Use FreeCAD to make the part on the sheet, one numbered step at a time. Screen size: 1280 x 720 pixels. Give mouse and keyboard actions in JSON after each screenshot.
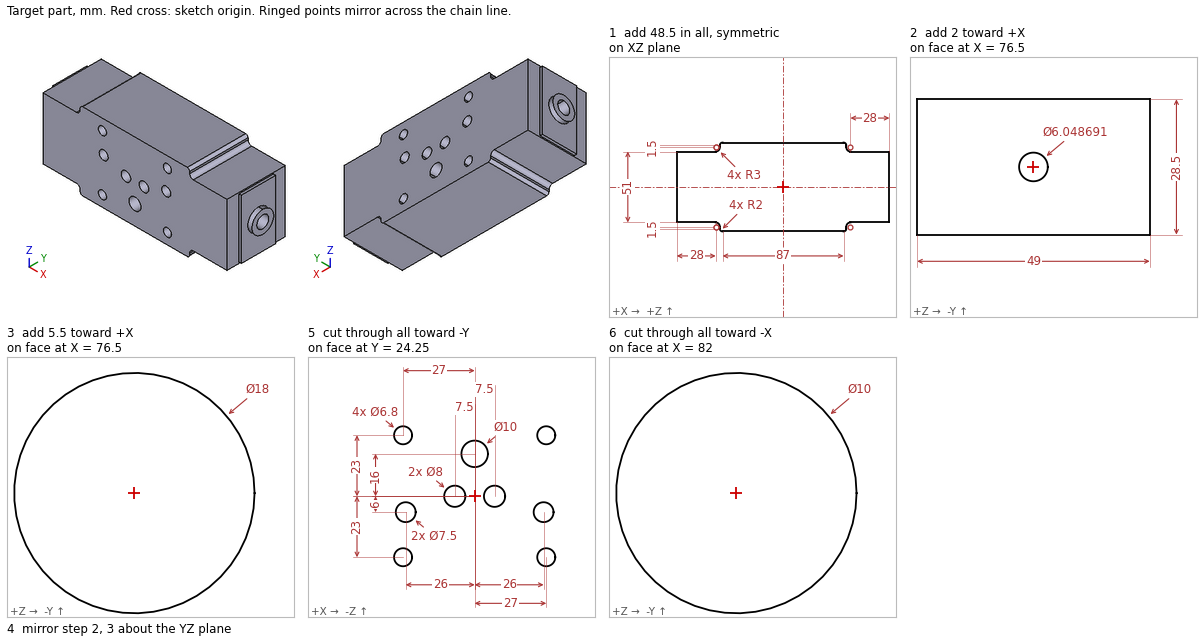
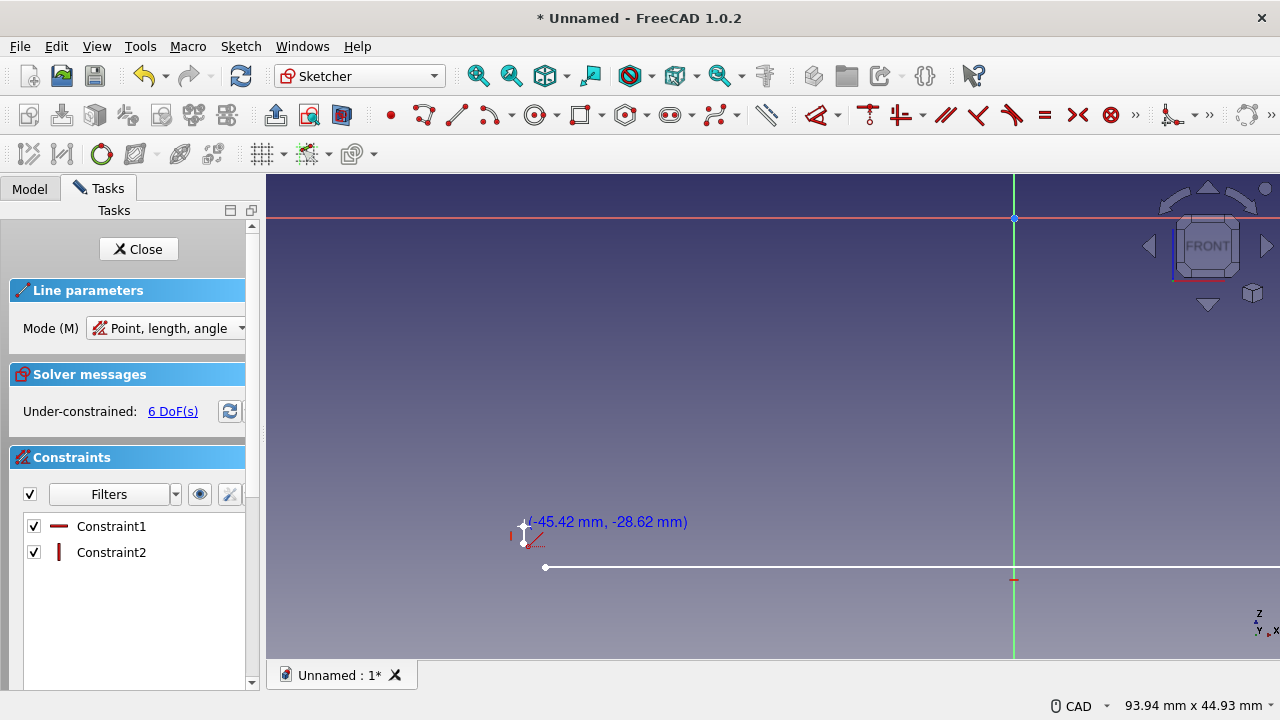
{"action": "left_click", "coordinate": [424, 116]}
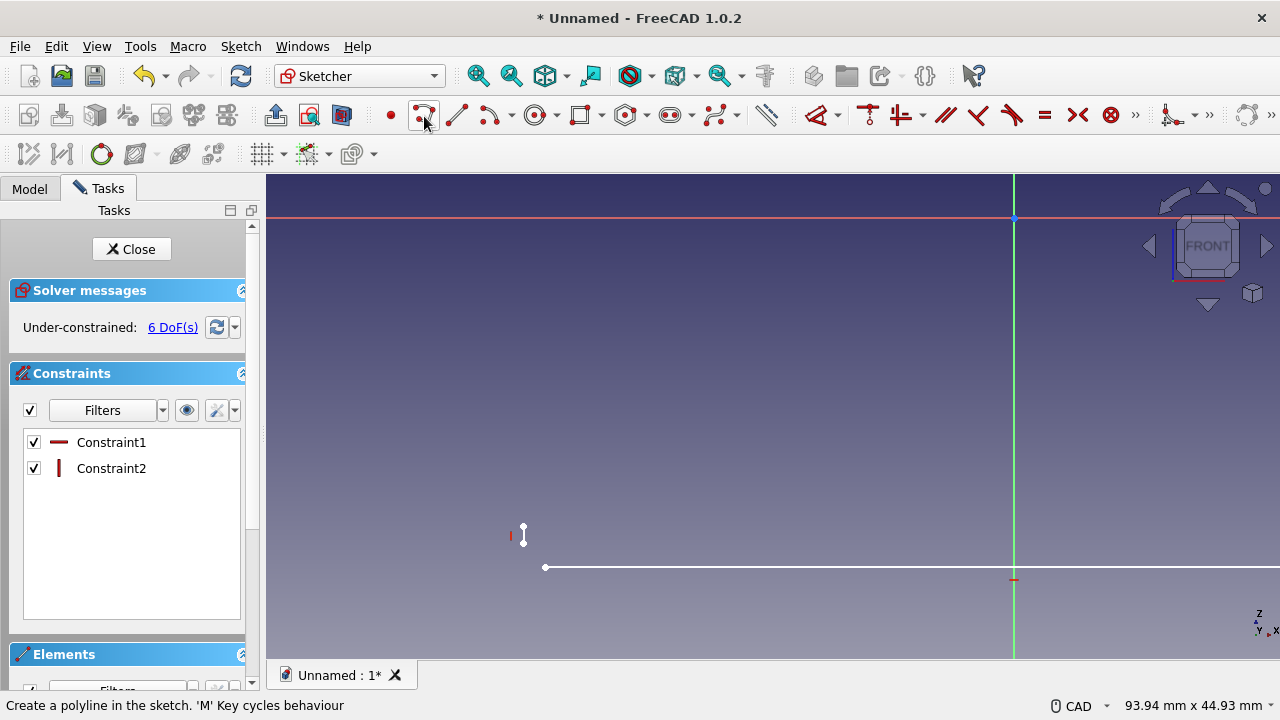
{"action": "left_click", "coordinate": [491, 493]}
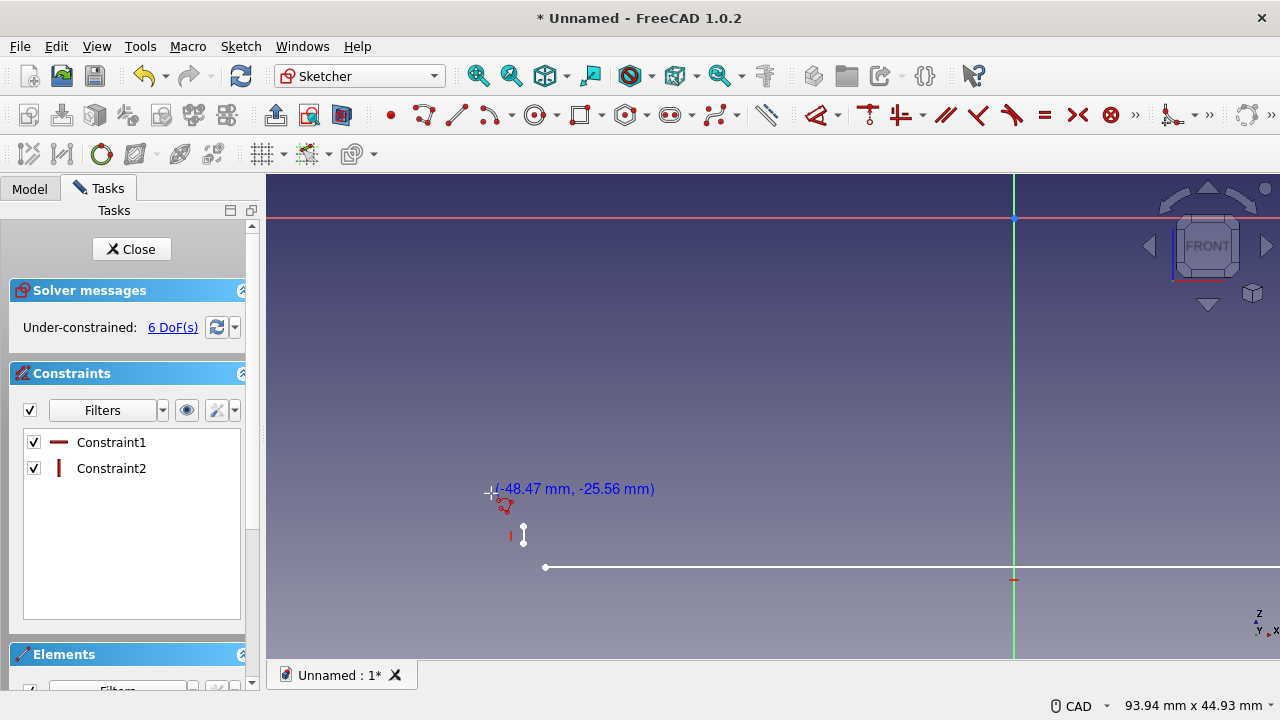
{"action": "scroll", "coordinate": [524, 532], "scroll_direction": "down", "scroll_amount": 5}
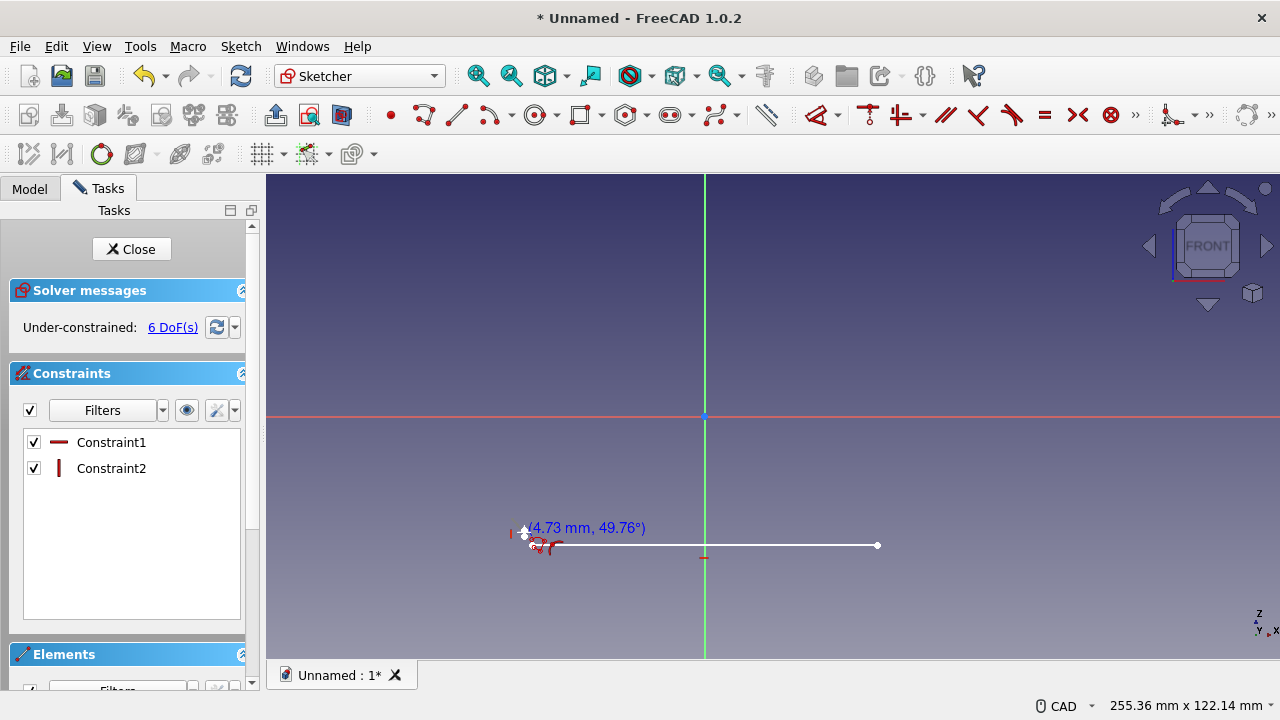
{"action": "left_click", "coordinate": [401, 518]}
{"action": "left_click", "coordinate": [401, 316]}
{"action": "left_click", "coordinate": [512, 316]}
{"action": "right_click", "coordinate": [512, 316]}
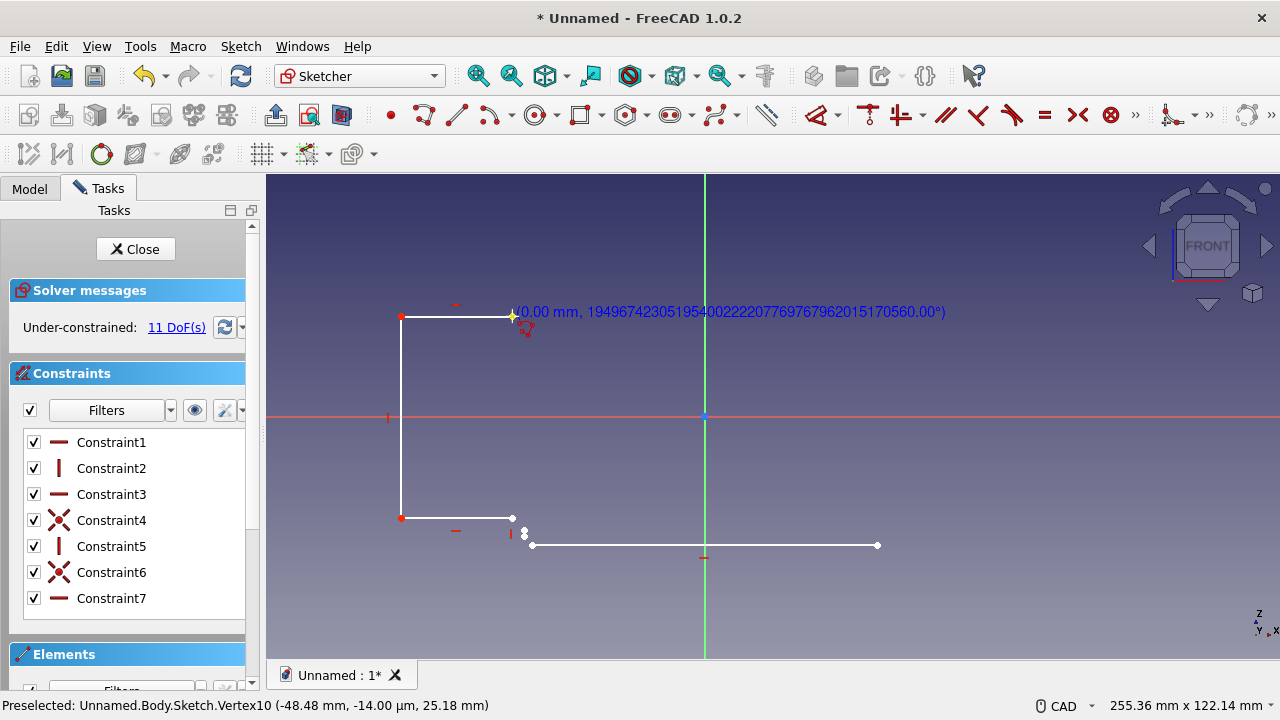
{"action": "left_click", "coordinate": [457, 116]}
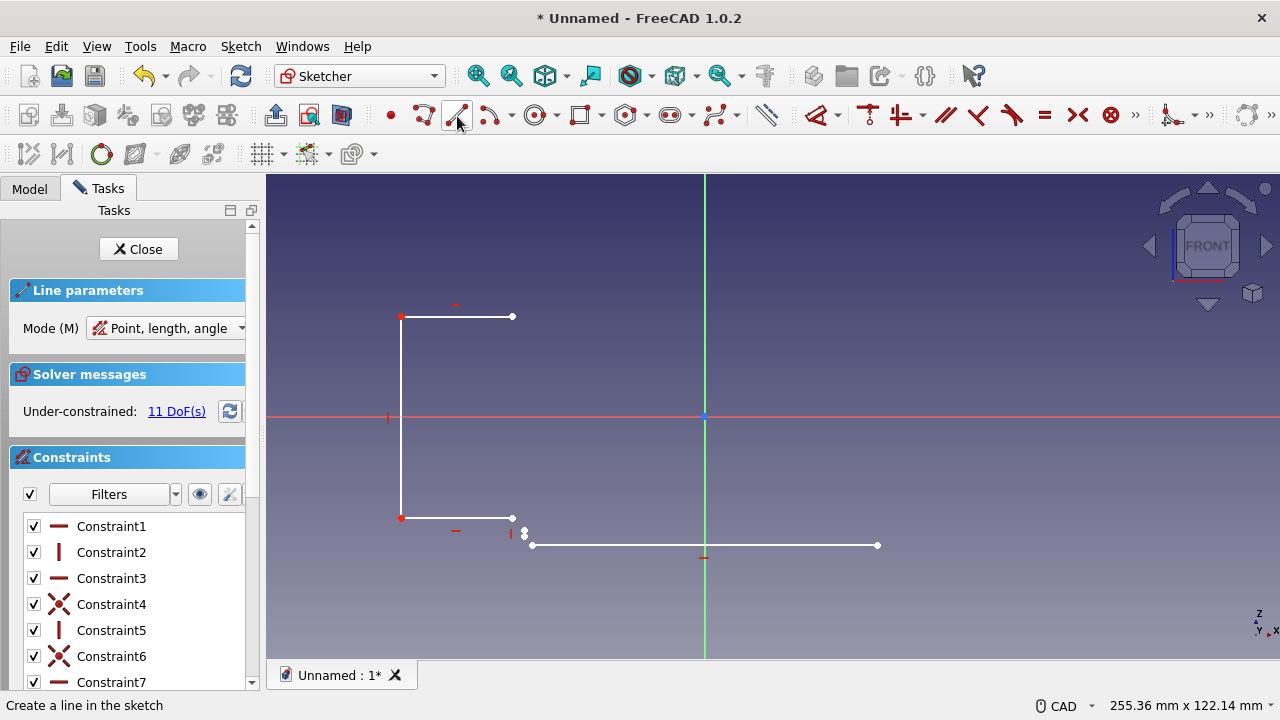
{"action": "left_click", "coordinate": [524, 304]}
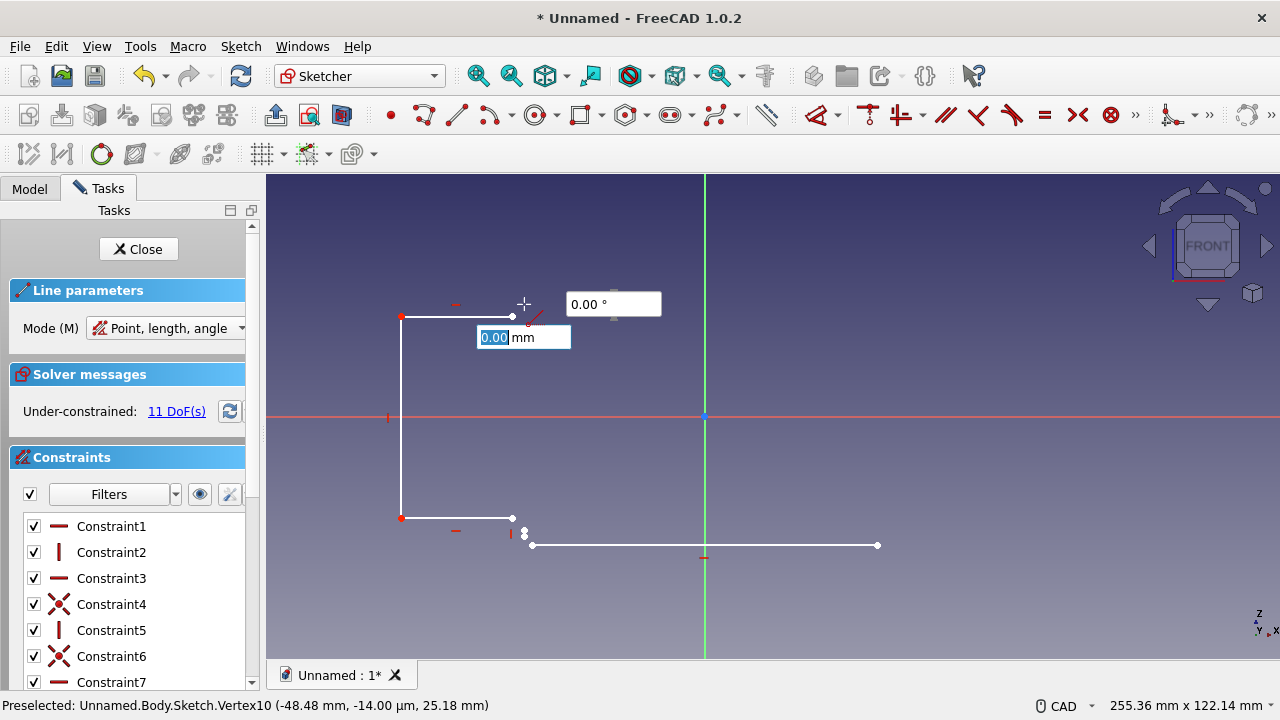
{"action": "scroll", "coordinate": [524, 298], "scroll_direction": "up", "scroll_amount": 5}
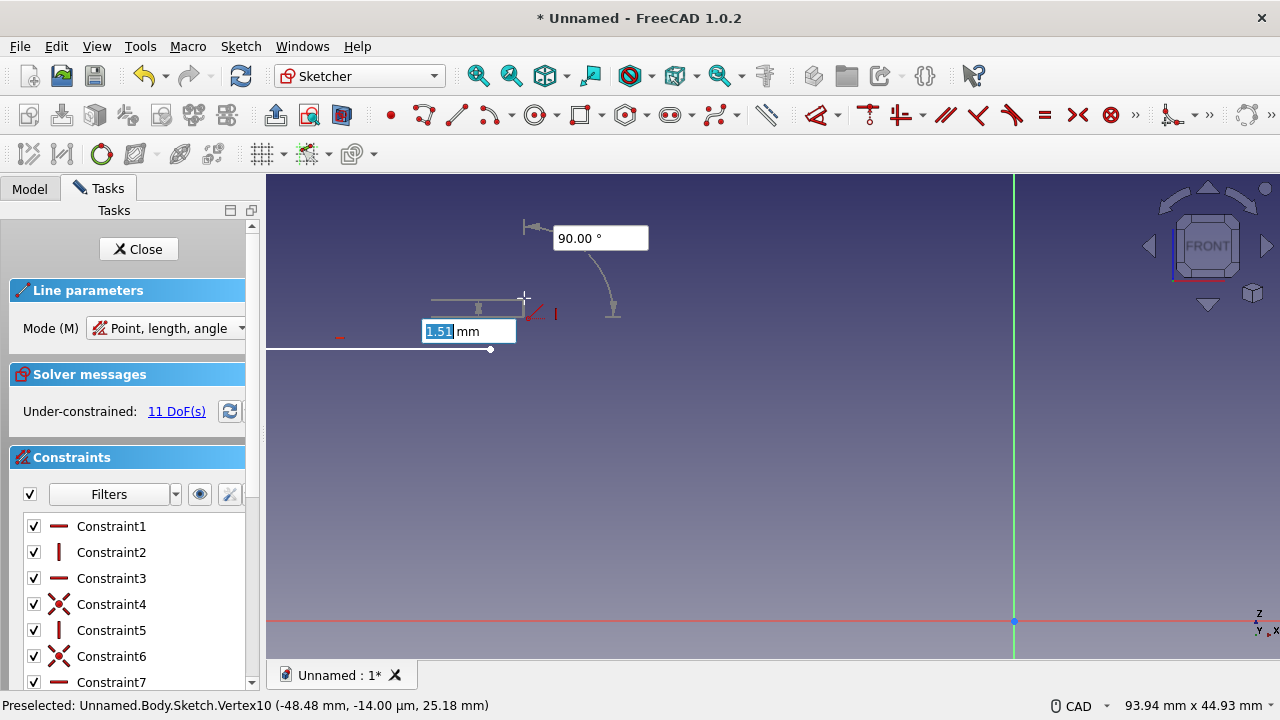
{"action": "left_click", "coordinate": [524, 297]}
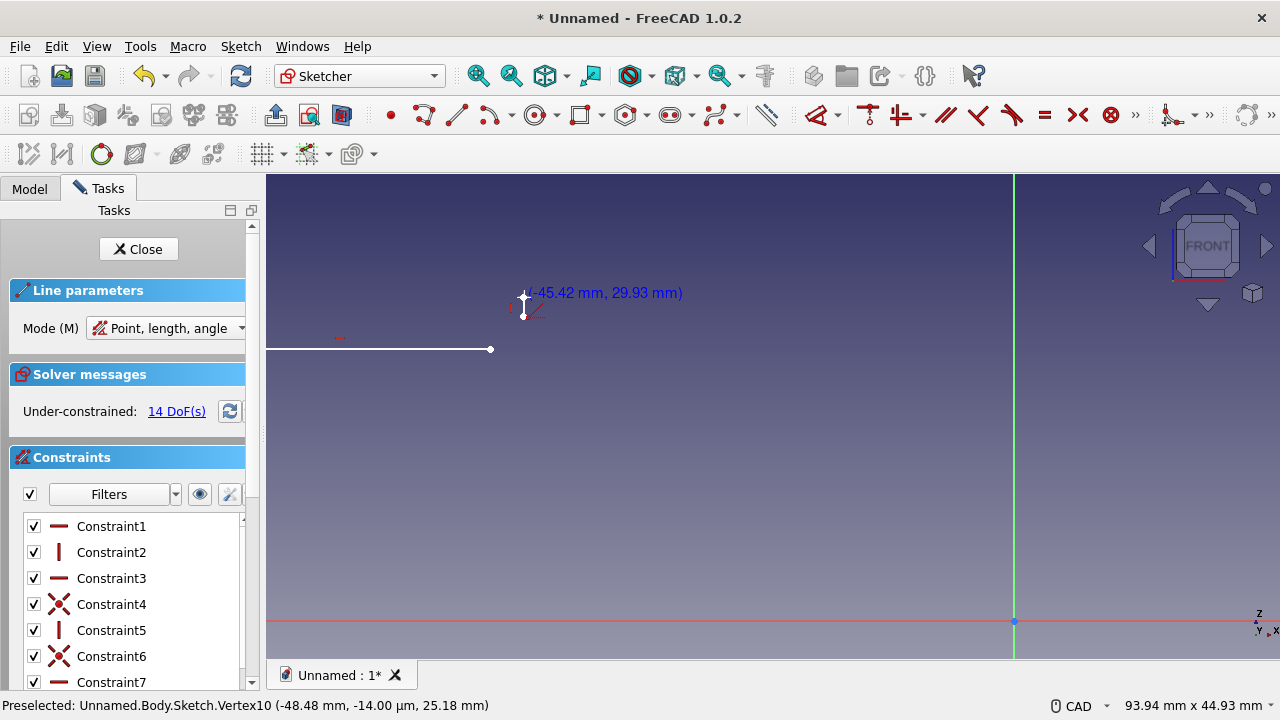
{"action": "left_click", "coordinate": [545, 276]}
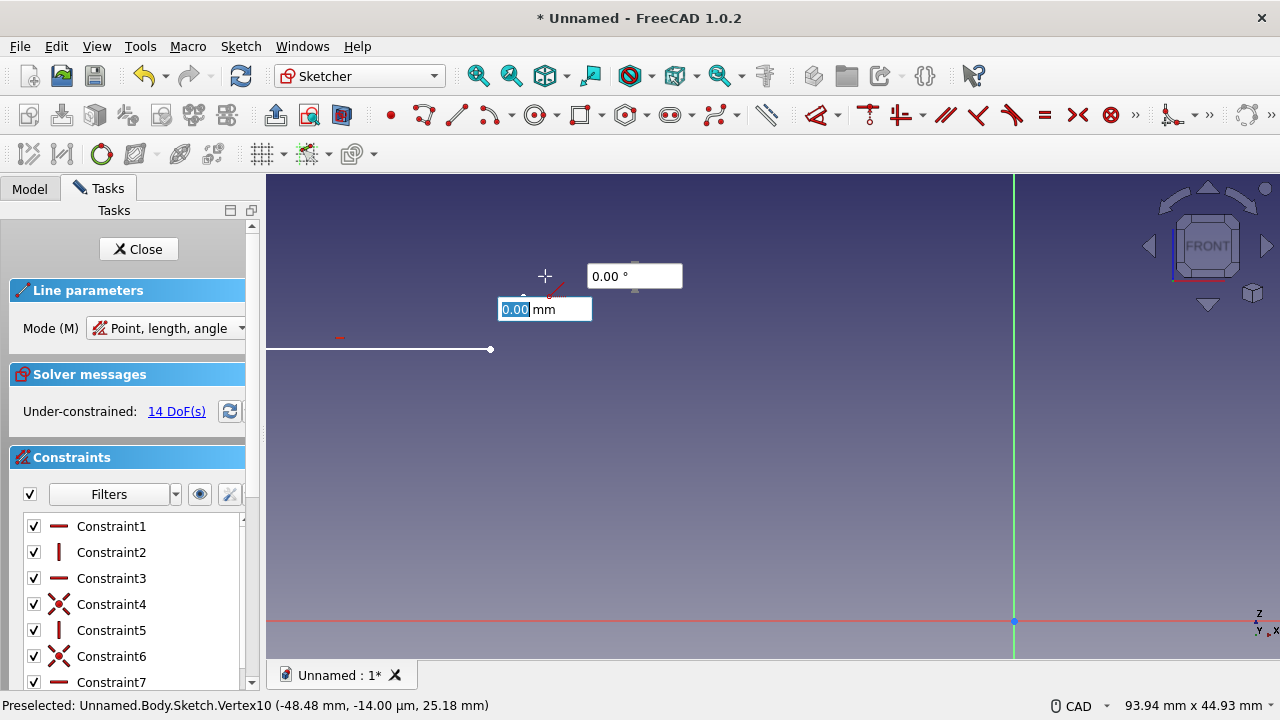
{"action": "scroll", "coordinate": [524, 297], "scroll_direction": "down", "scroll_amount": 5}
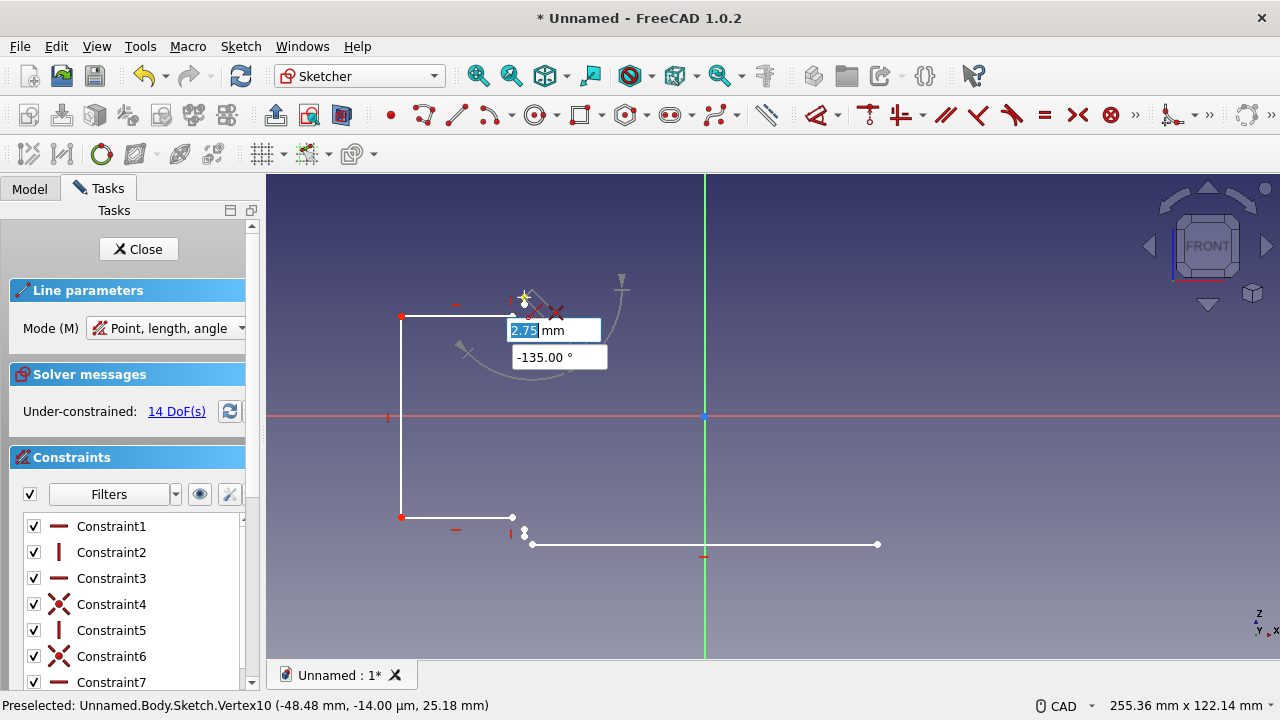
{"action": "left_click", "coordinate": [877, 289]}